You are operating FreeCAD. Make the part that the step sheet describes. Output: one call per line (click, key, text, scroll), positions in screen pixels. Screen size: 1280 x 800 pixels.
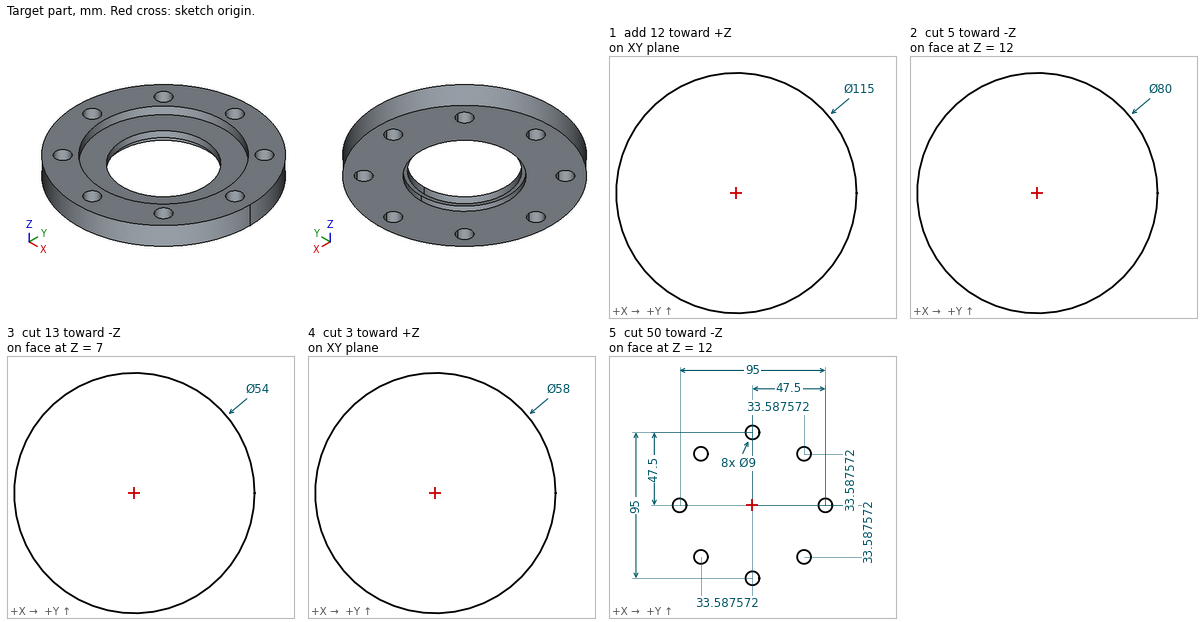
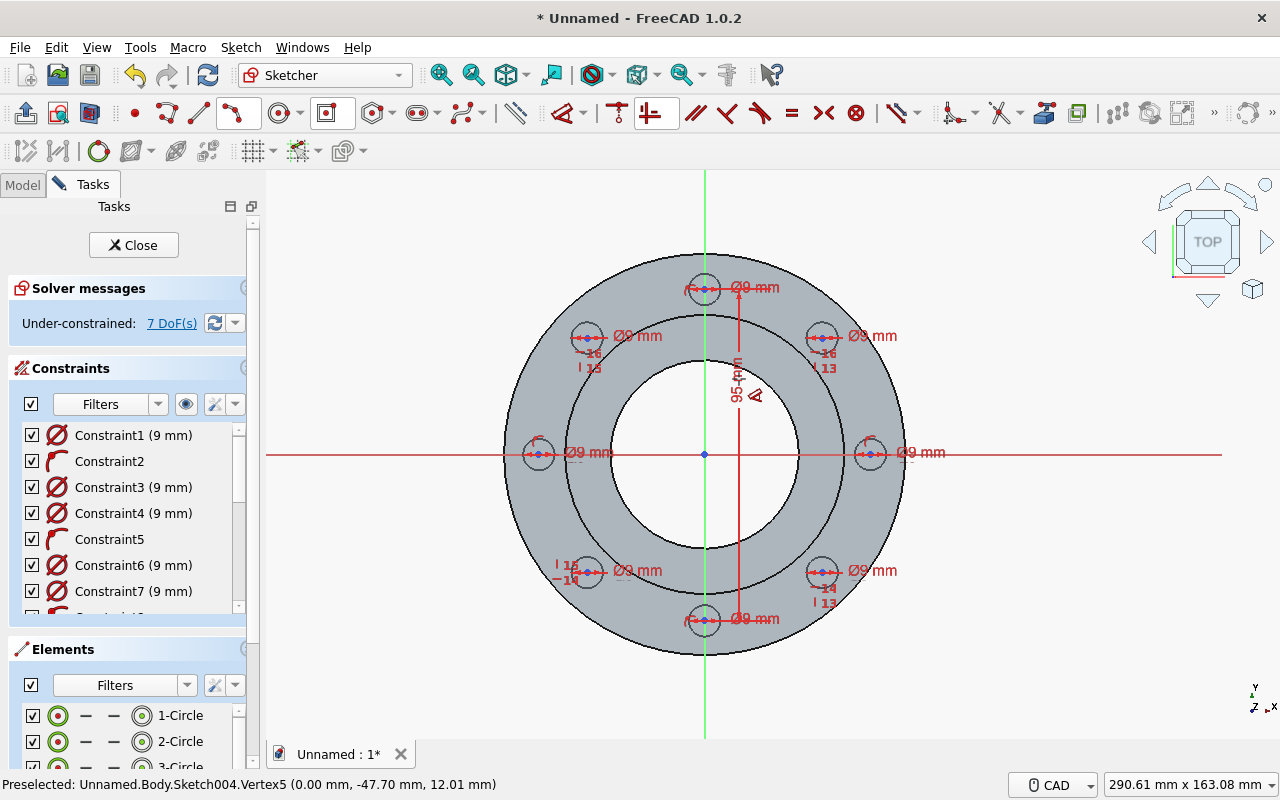
click(870, 454)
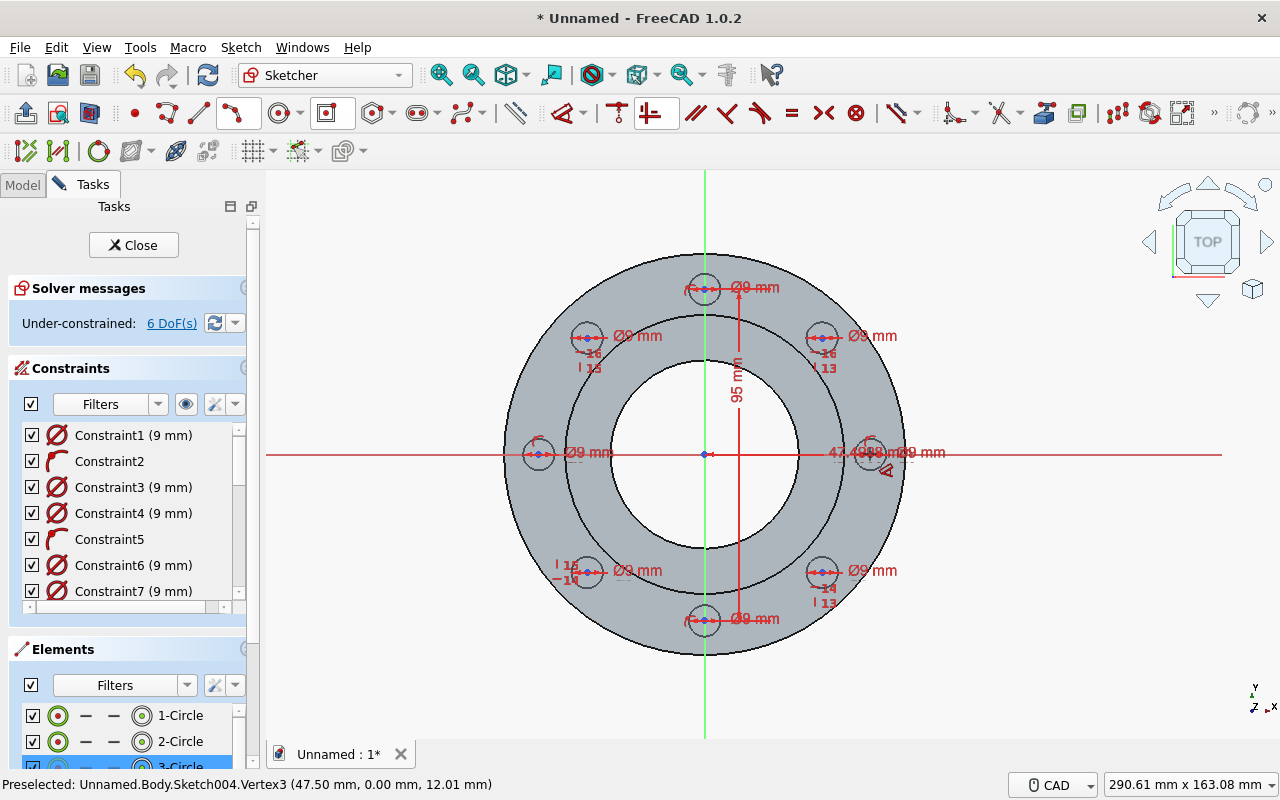
click(539, 454)
click(628, 488)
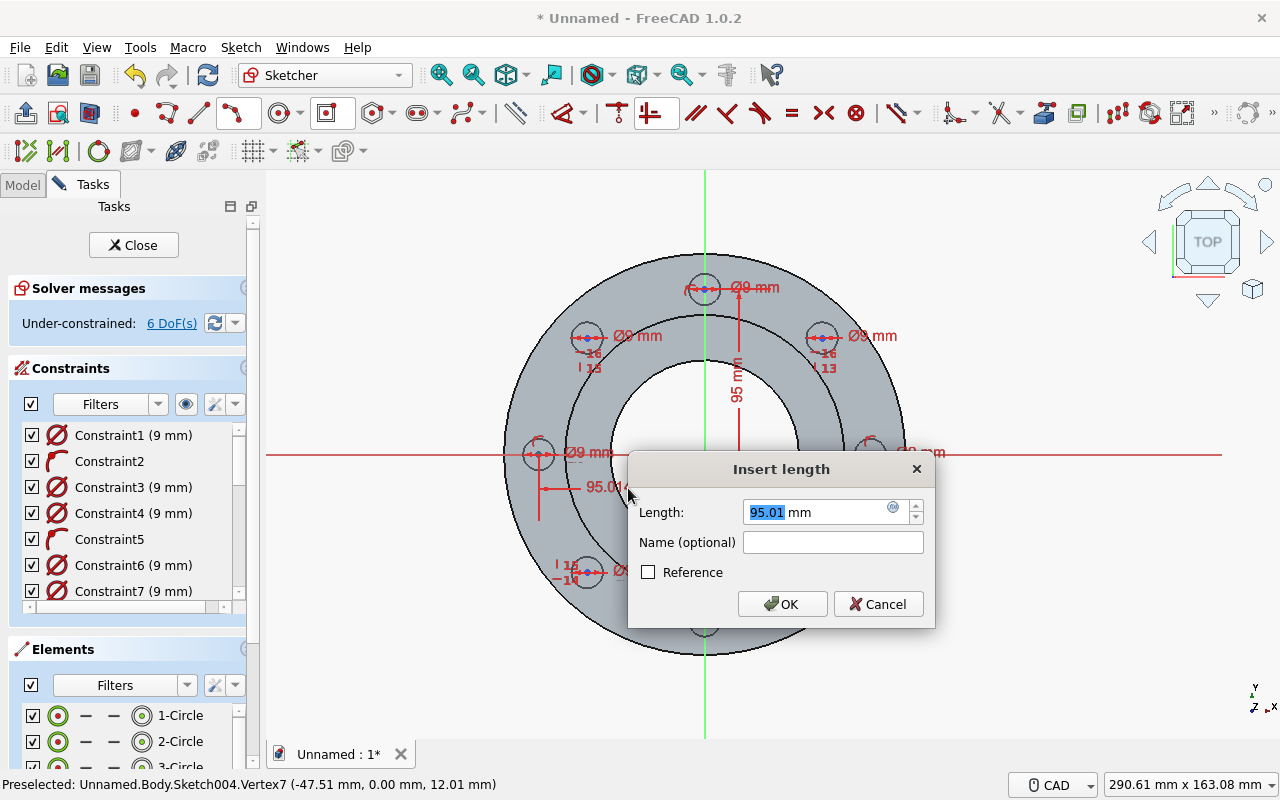
text(95)
key(Return)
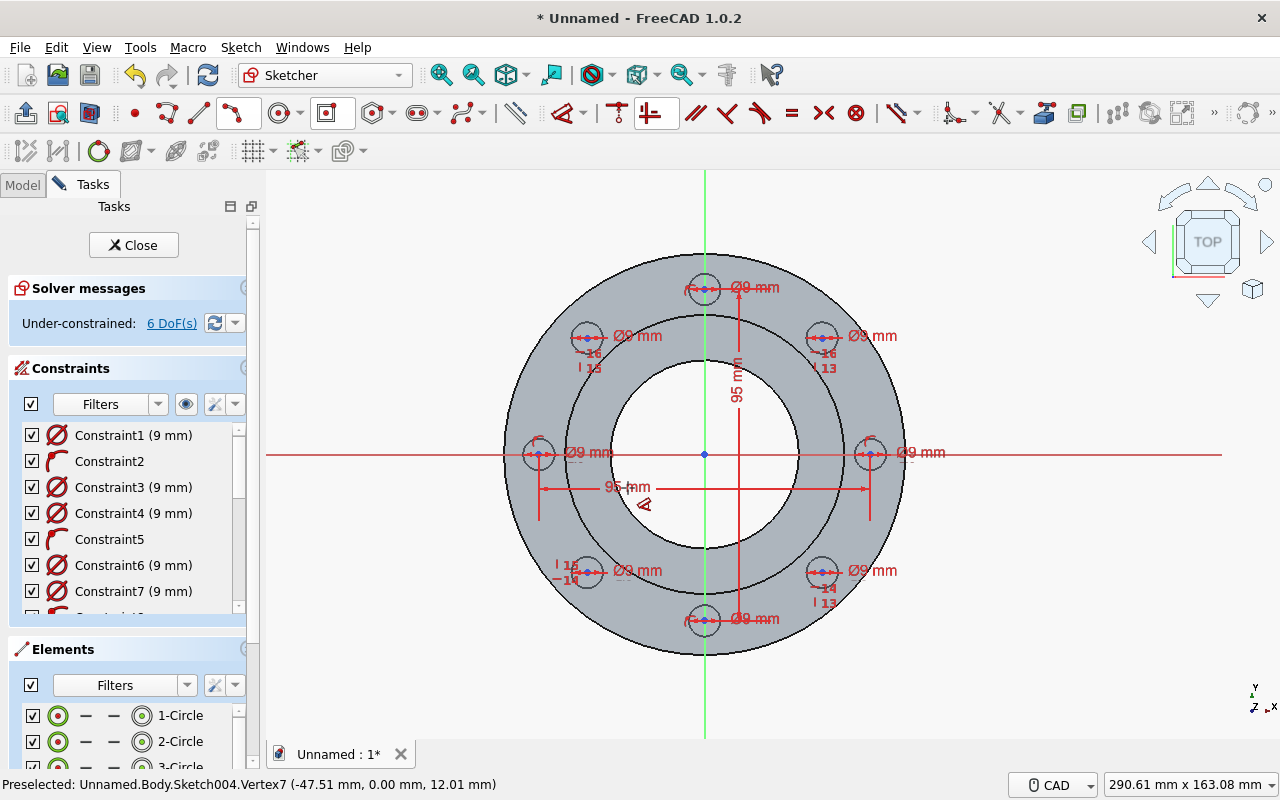
click(705, 289)
click(739, 334)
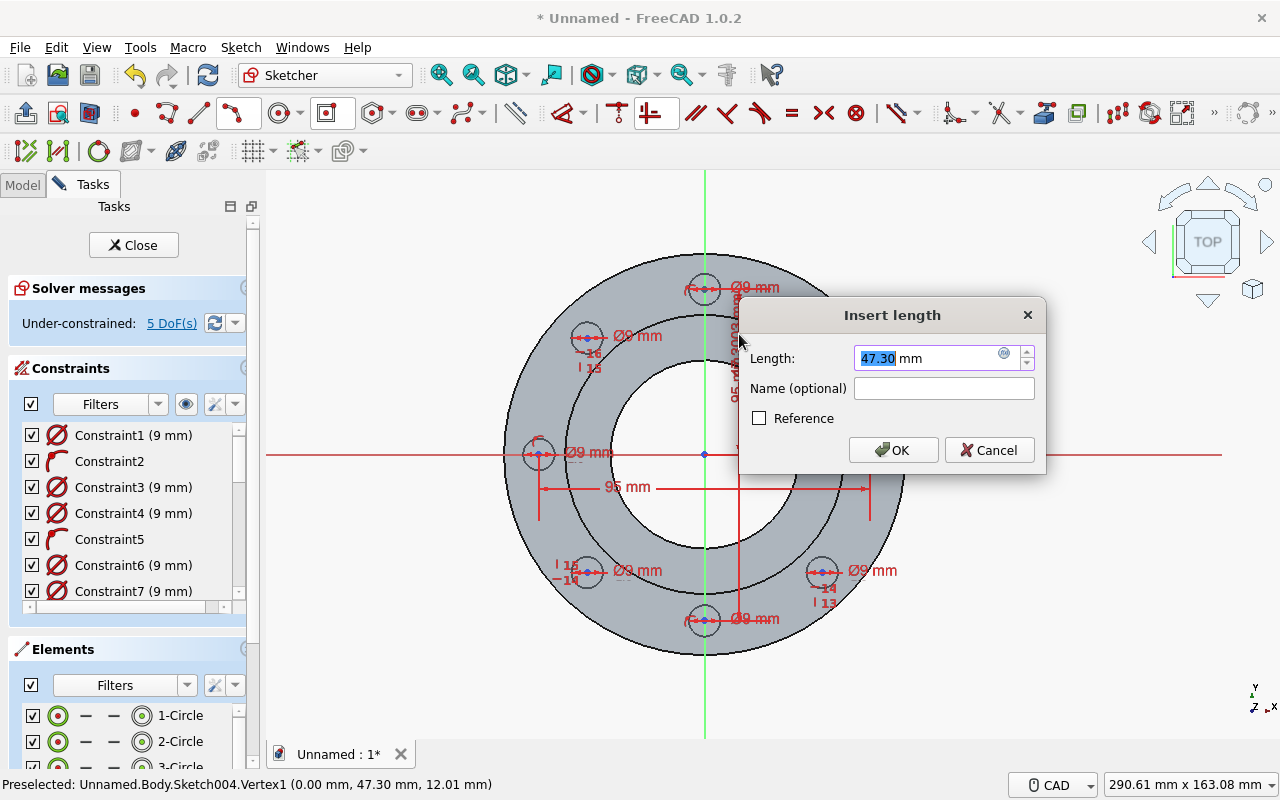
text(47.5)
key(Return)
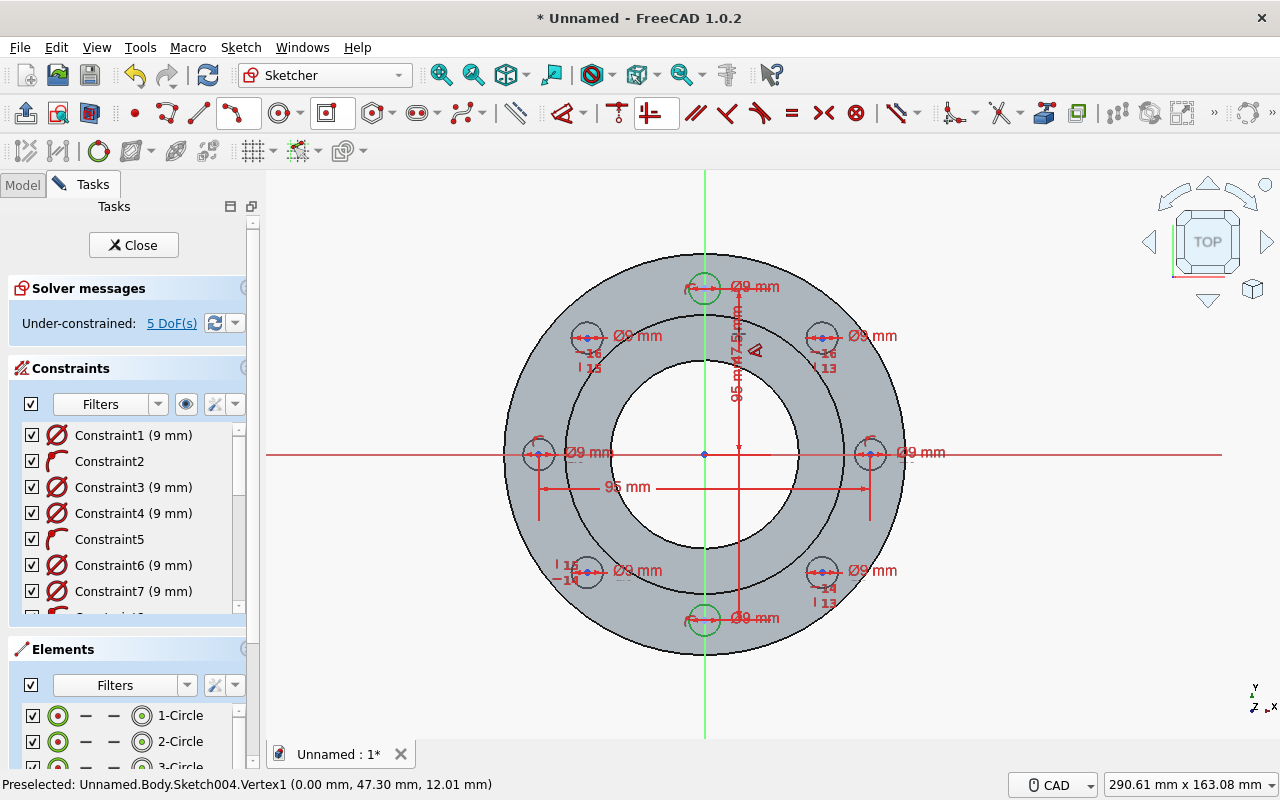
click(870, 454)
click(788, 488)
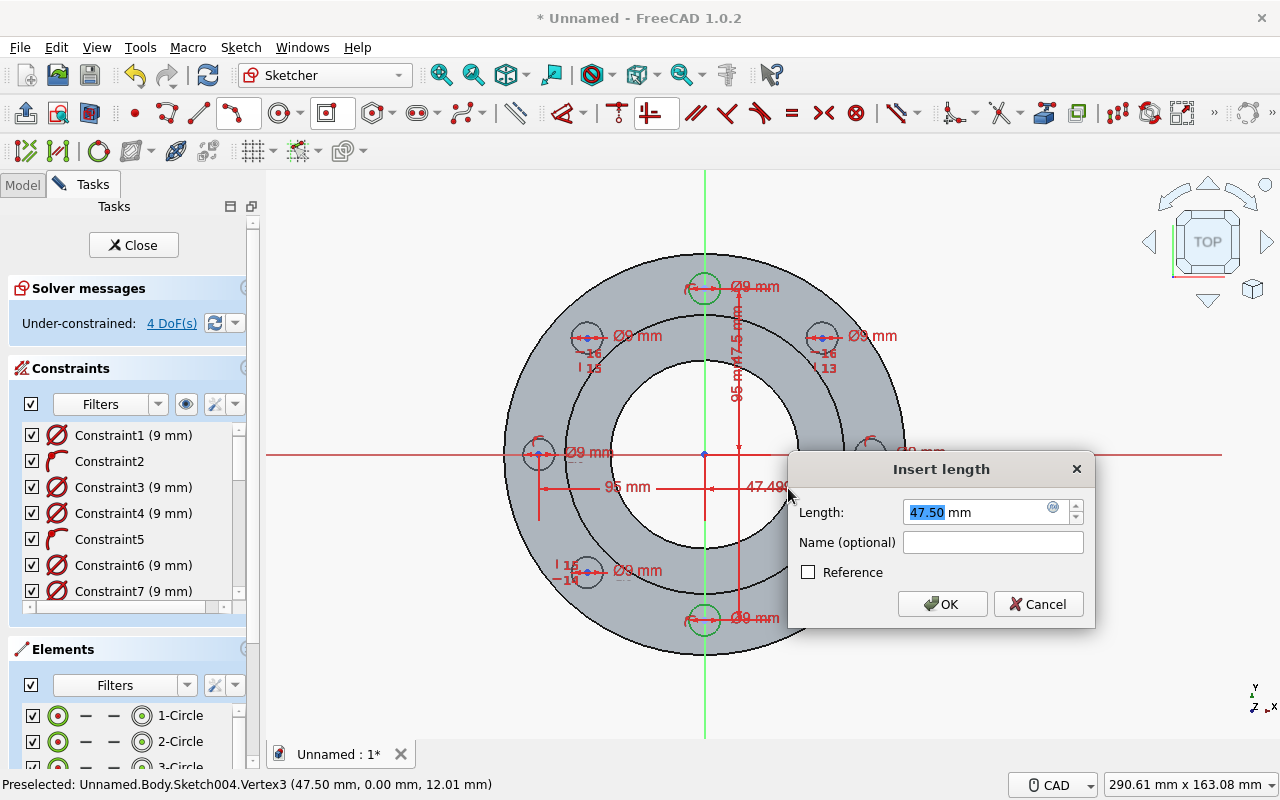
text(47.5)
key(Return)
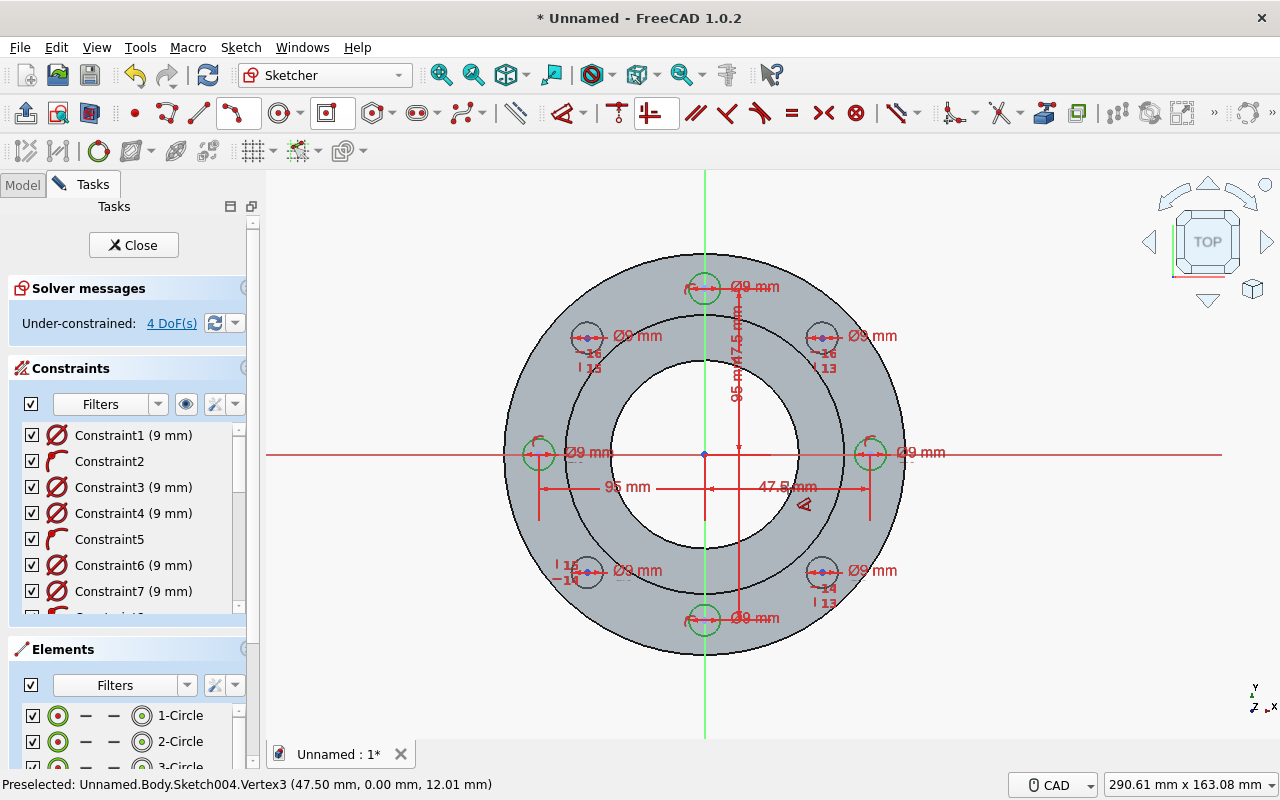
click(822, 338)
click(763, 304)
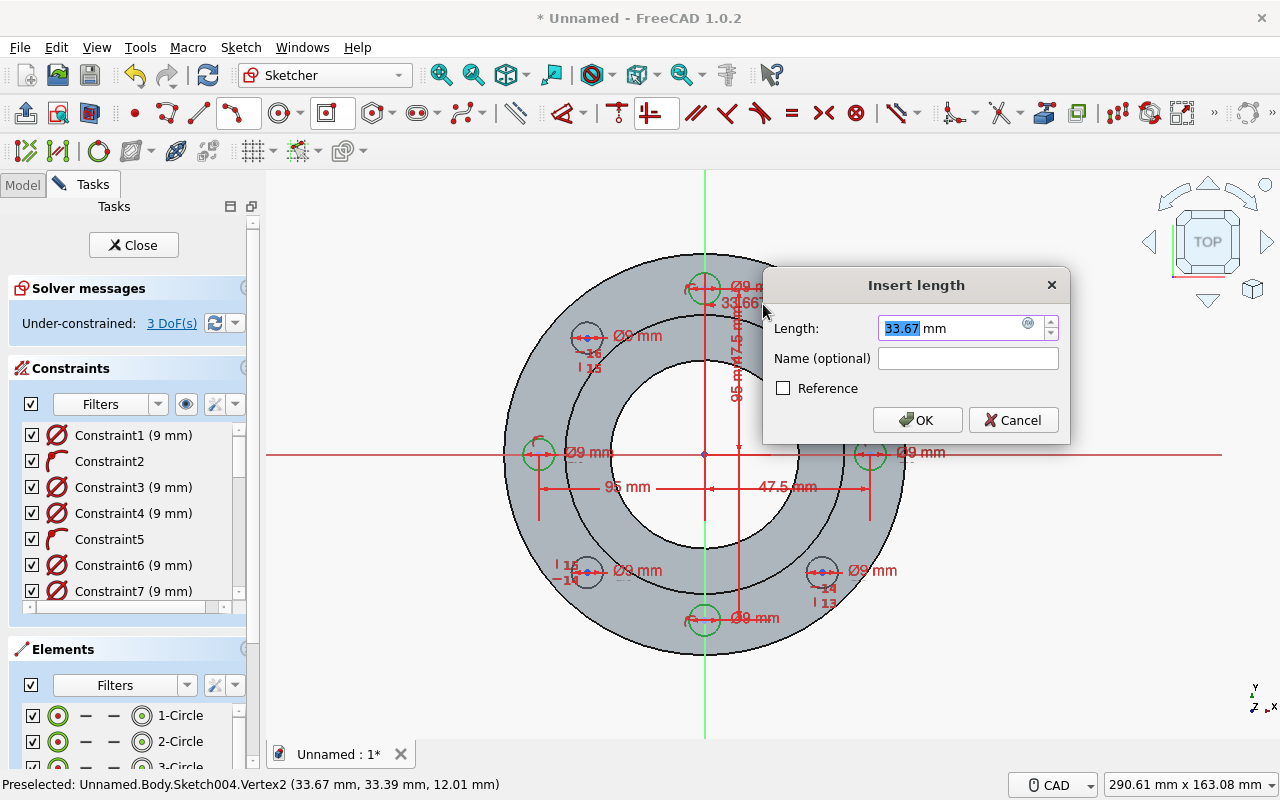
text(33.587572)
key(Return)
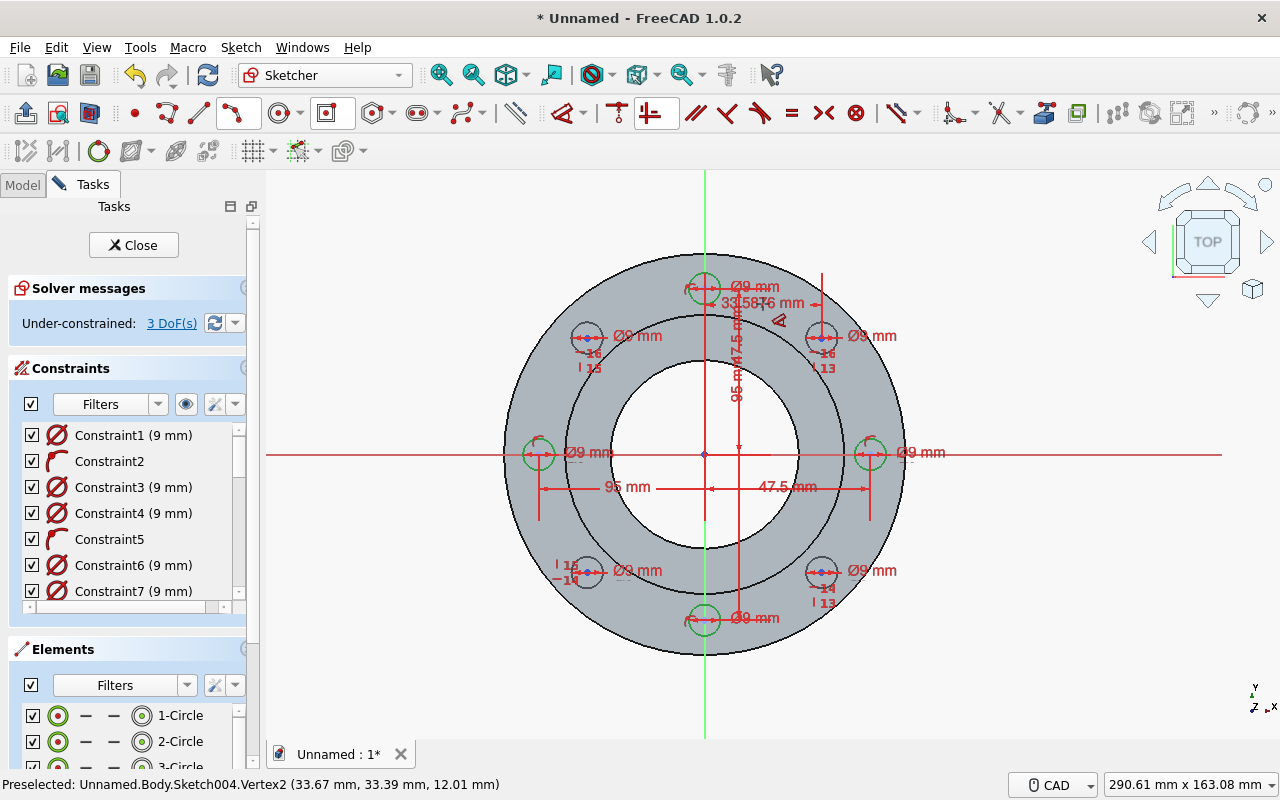
click(822, 338)
click(856, 396)